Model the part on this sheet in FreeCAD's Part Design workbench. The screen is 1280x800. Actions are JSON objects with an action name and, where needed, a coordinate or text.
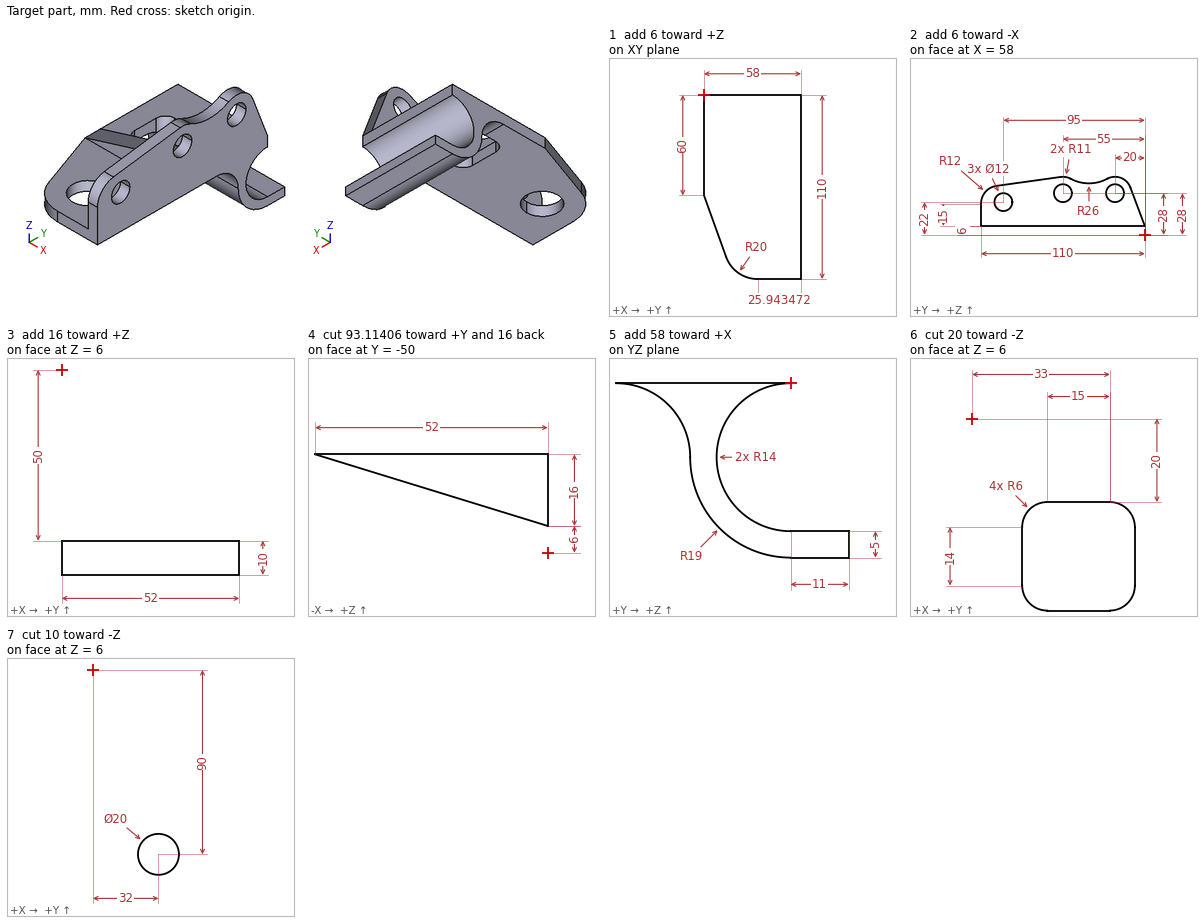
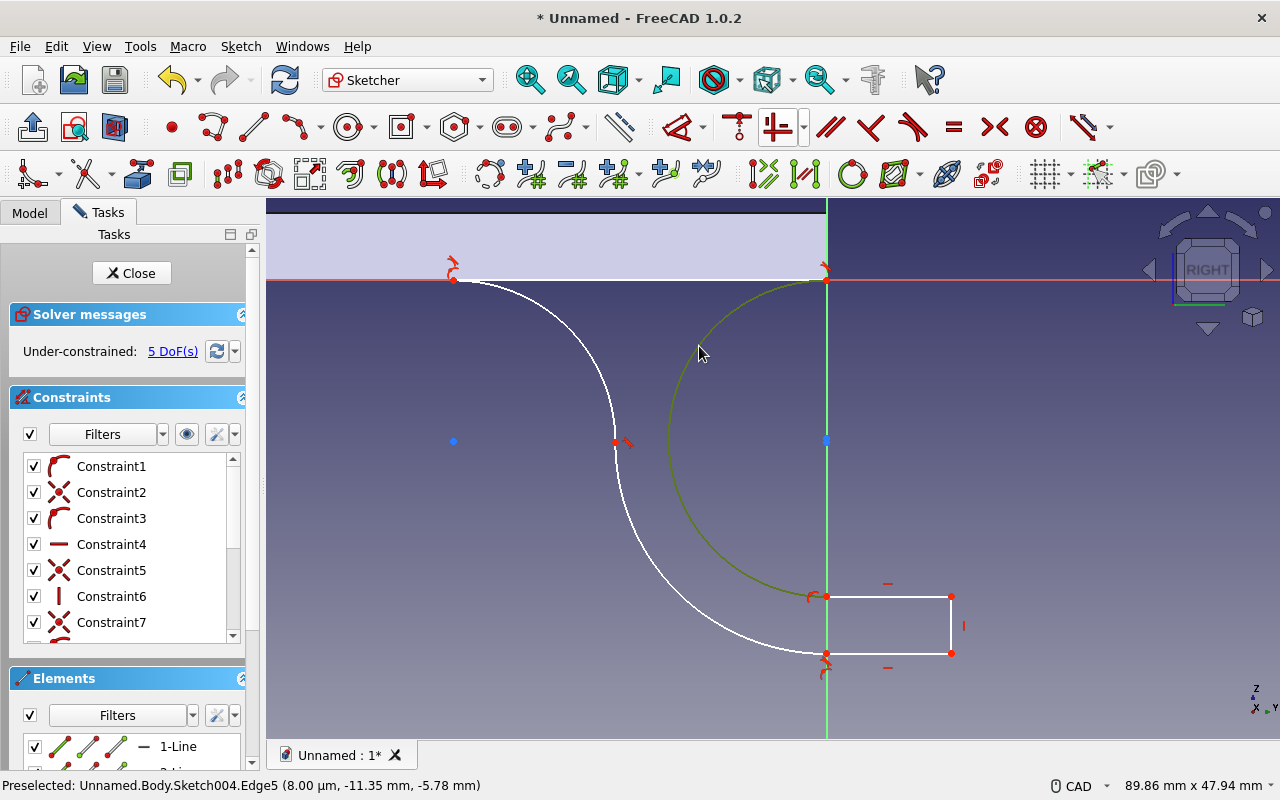
{"action": "left_click", "coordinate": [598, 369]}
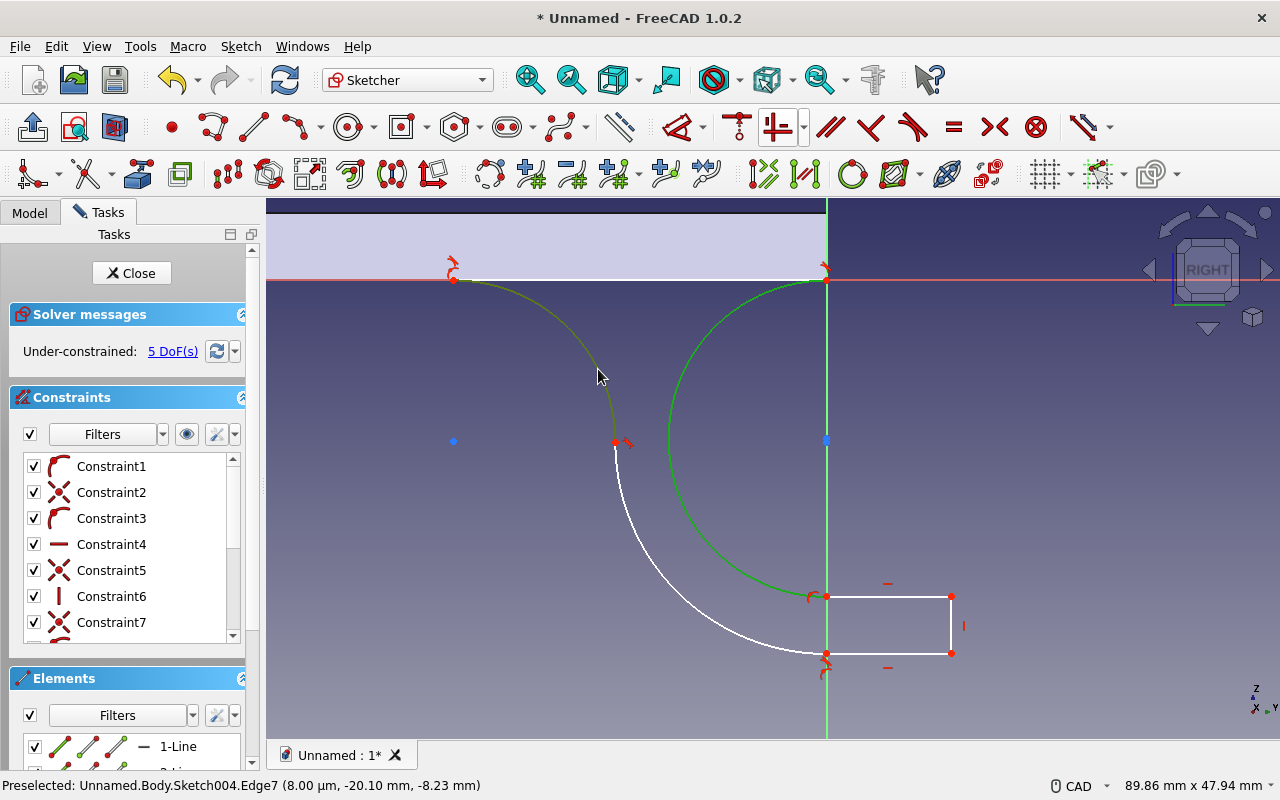
{"action": "left_click", "coordinate": [954, 128]}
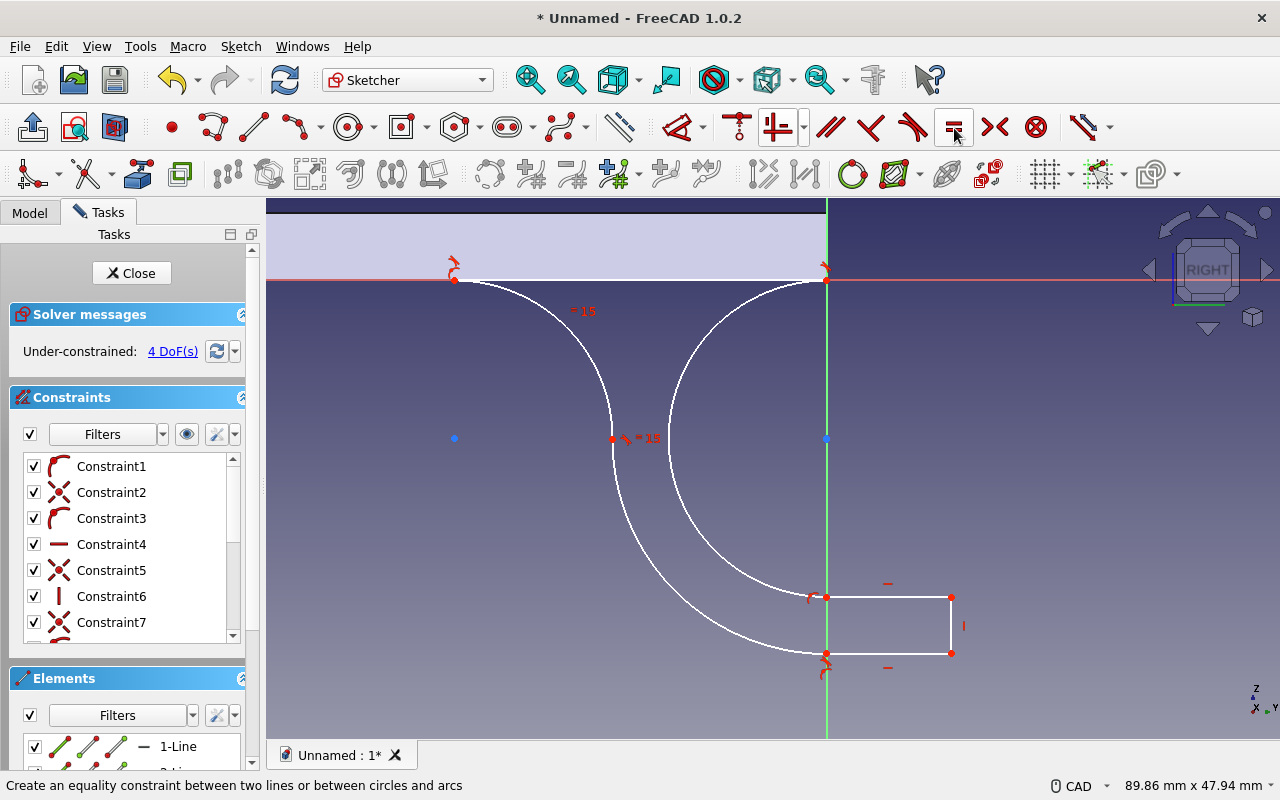
{"action": "key", "text": "d"}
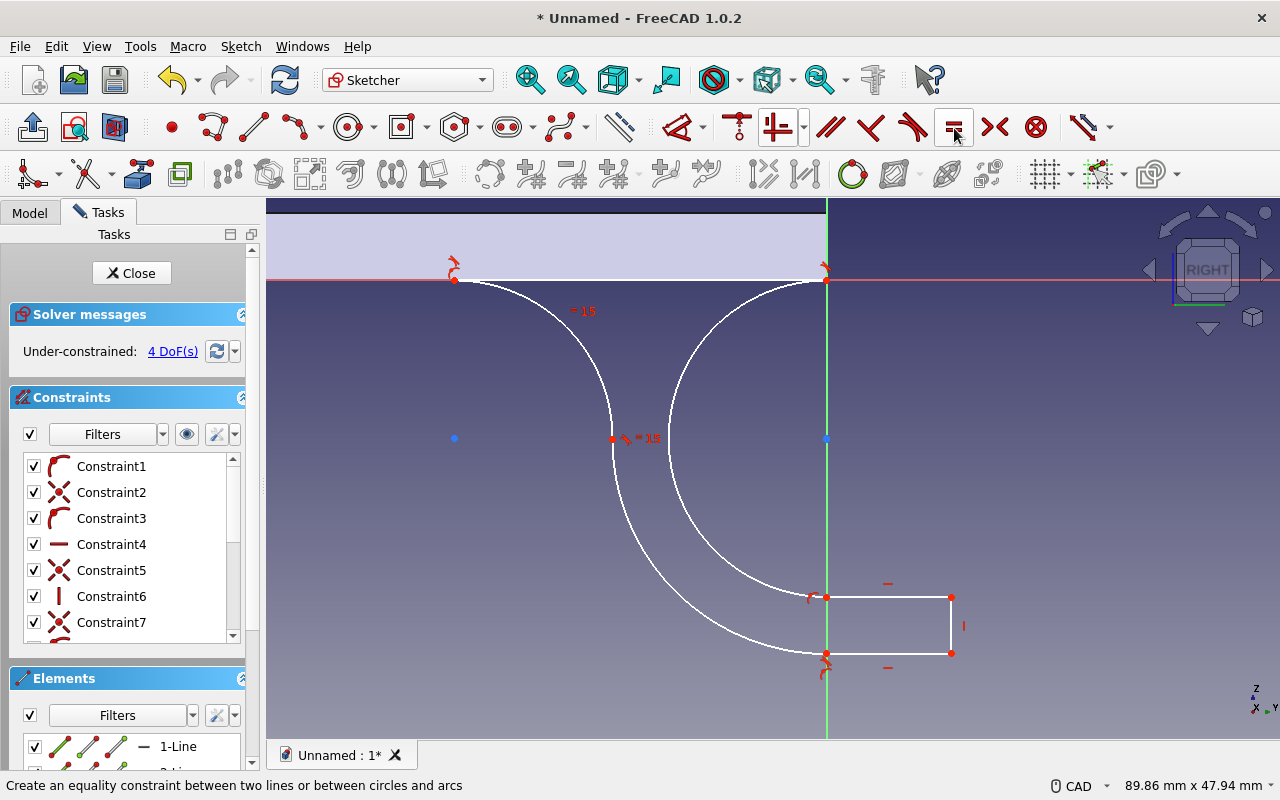
{"action": "left_click", "coordinate": [699, 346]}
{"action": "left_click", "coordinate": [673, 327]}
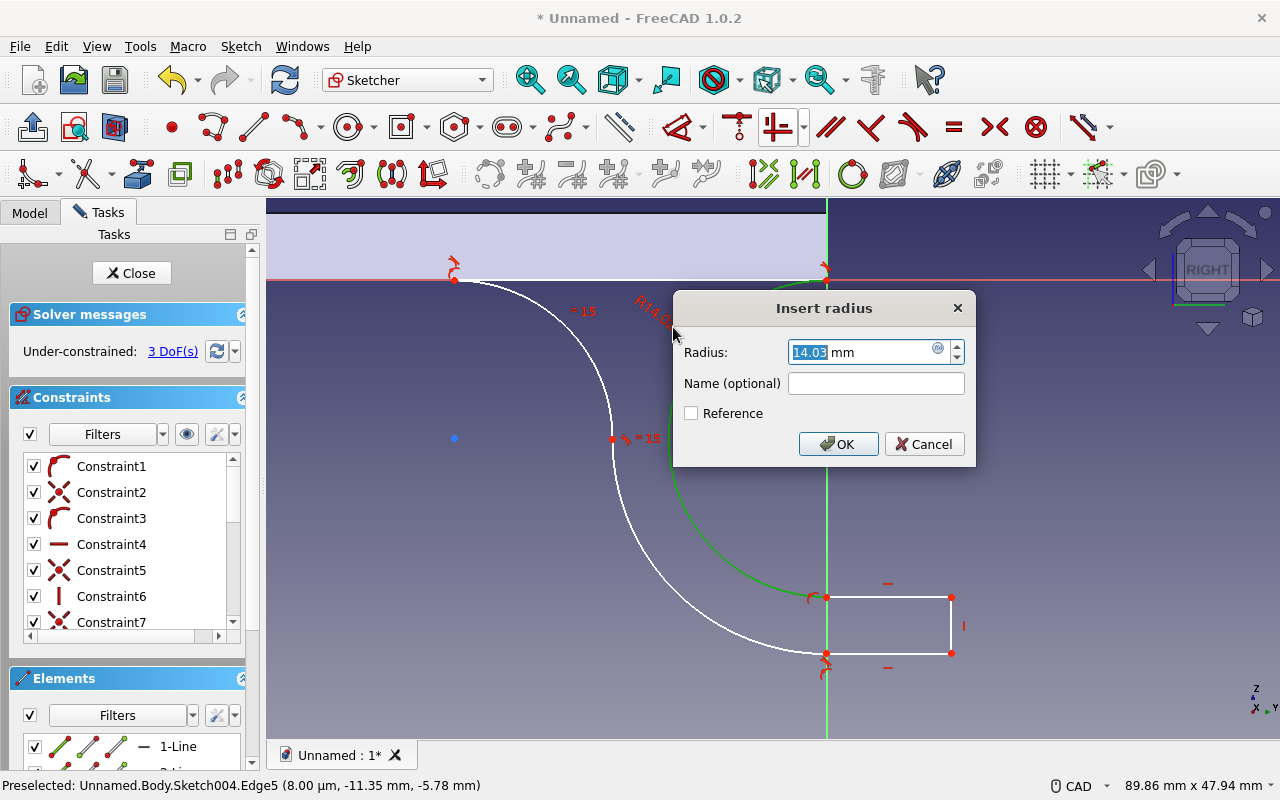
{"action": "type", "text": "14"}
{"action": "key", "text": "Return"}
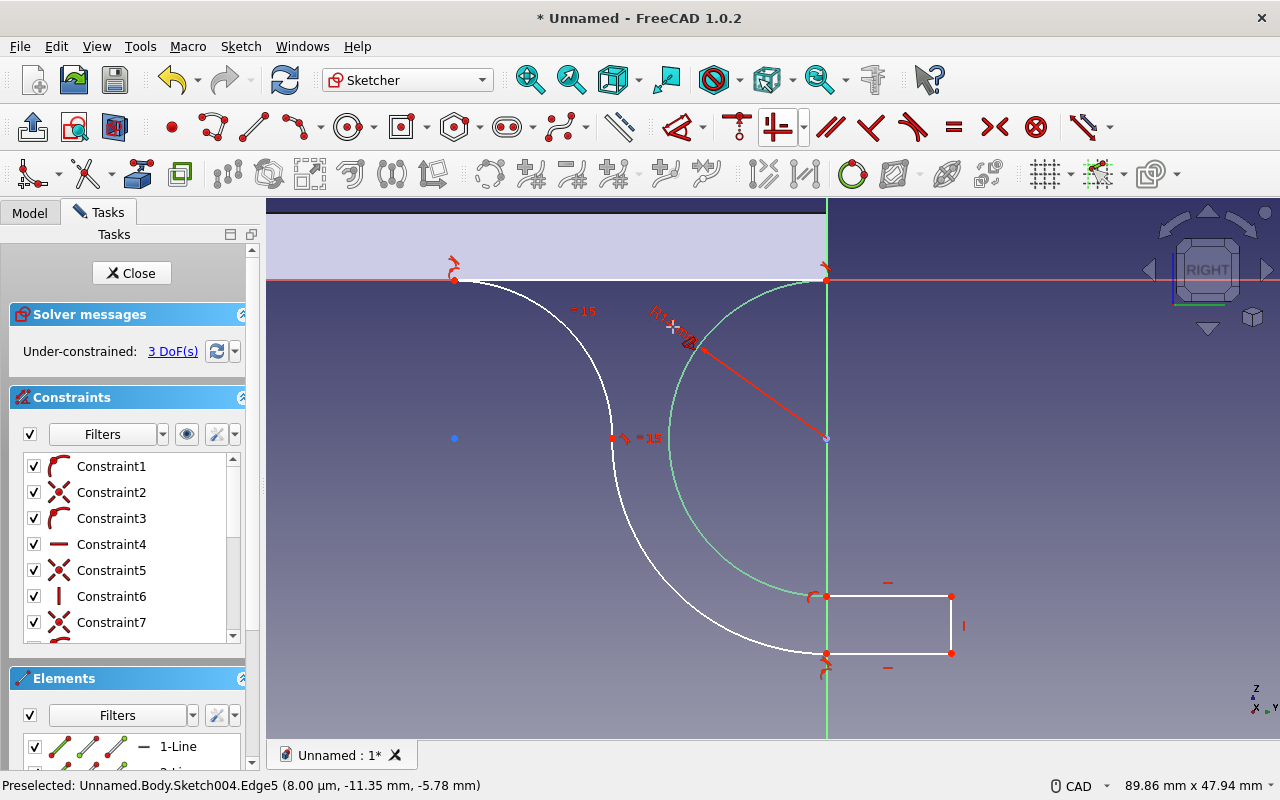
{"action": "left_click", "coordinate": [635, 536]}
{"action": "left_click", "coordinate": [606, 550]}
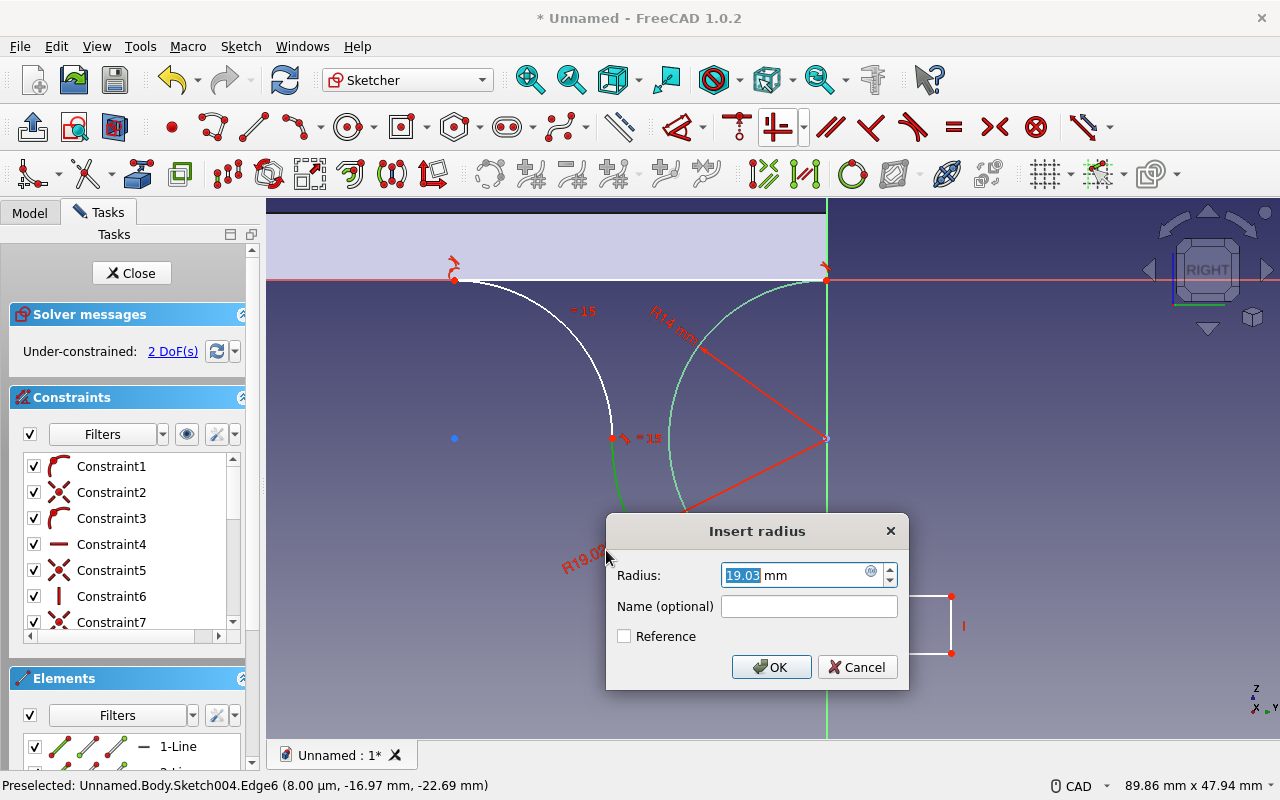
{"action": "type", "text": "19"}
{"action": "key", "text": "Return"}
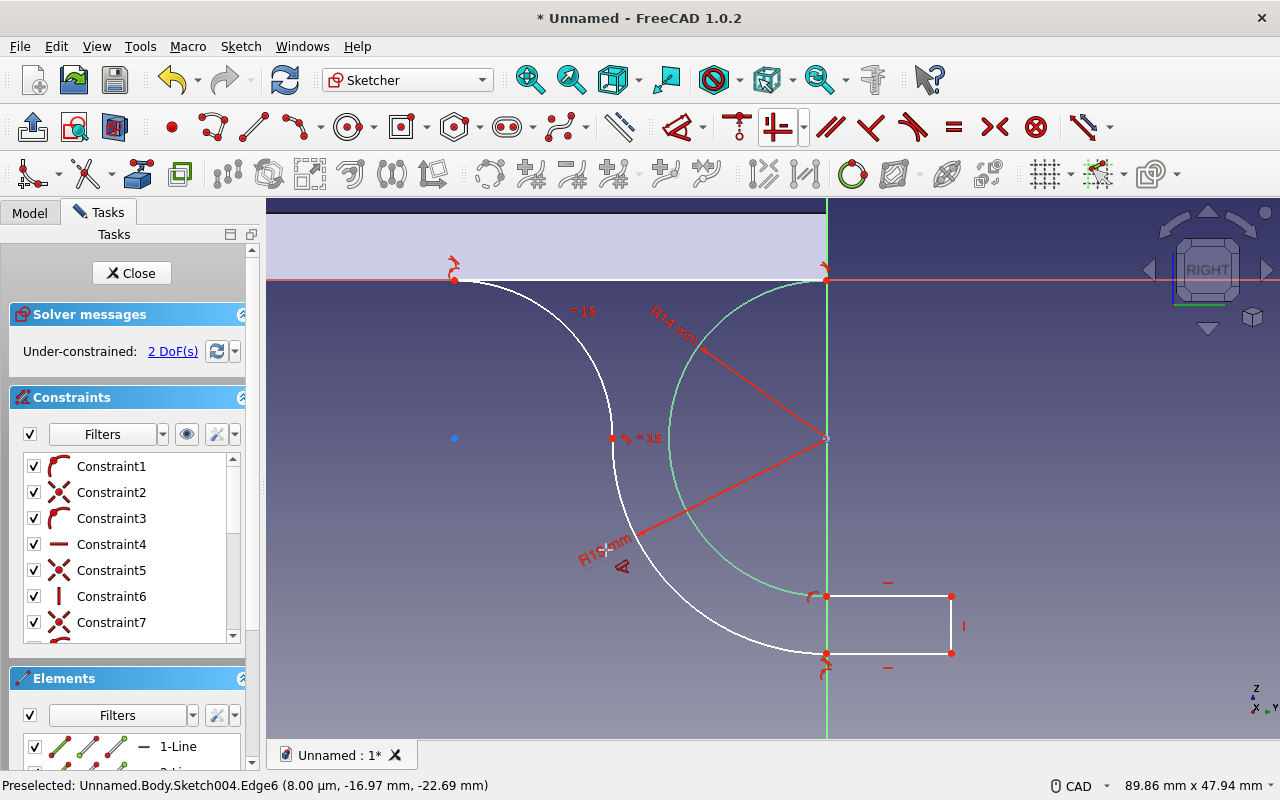
{"action": "left_click", "coordinate": [951, 614]}
{"action": "left_click", "coordinate": [985, 625]}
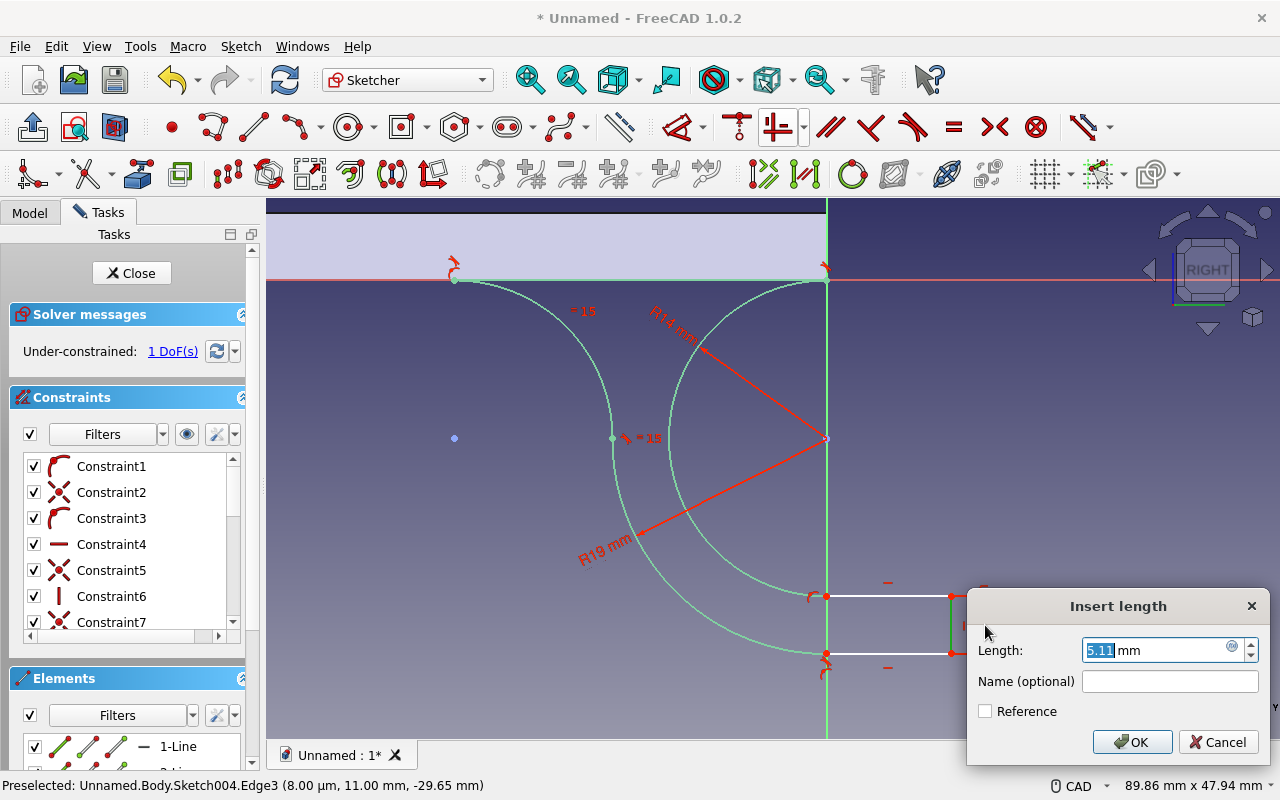
{"action": "type", "text": "5"}
{"action": "key", "text": "Return"}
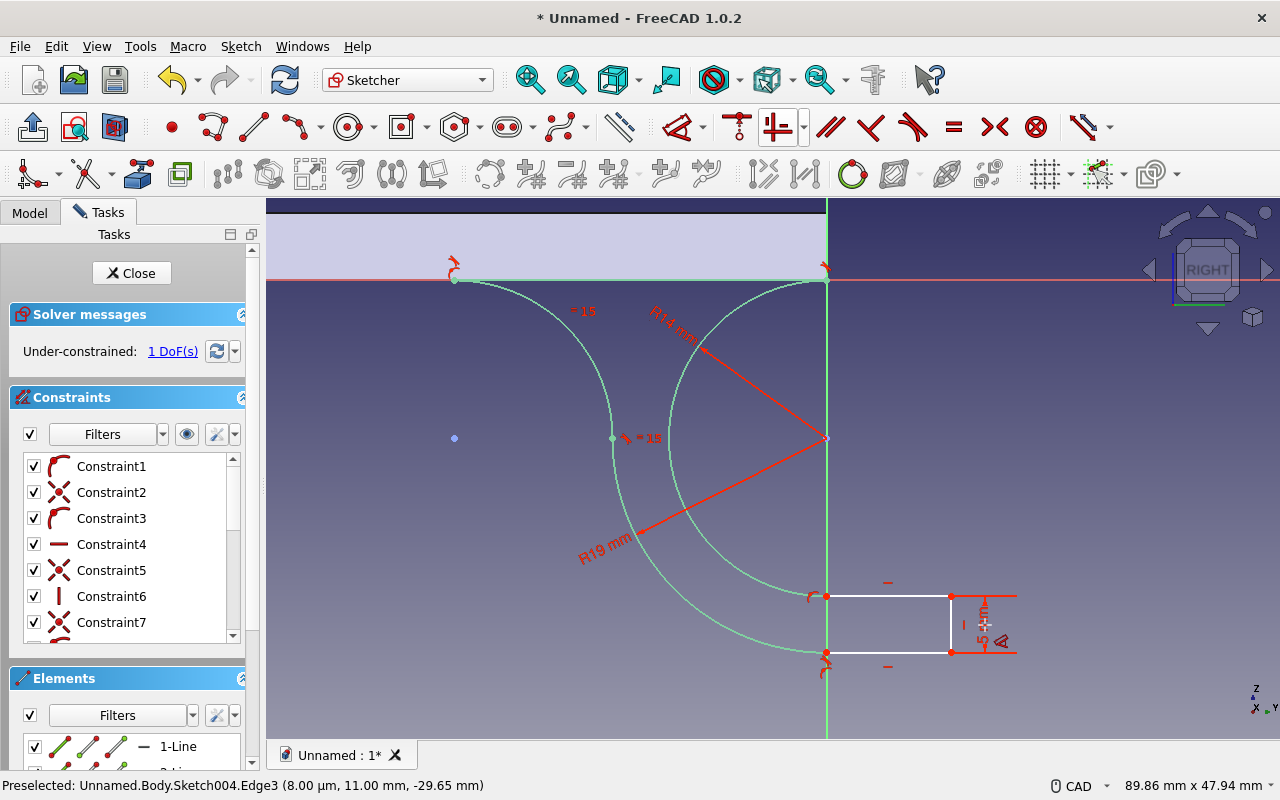
{"action": "left_click", "coordinate": [864, 596]}
{"action": "left_click", "coordinate": [889, 630]}